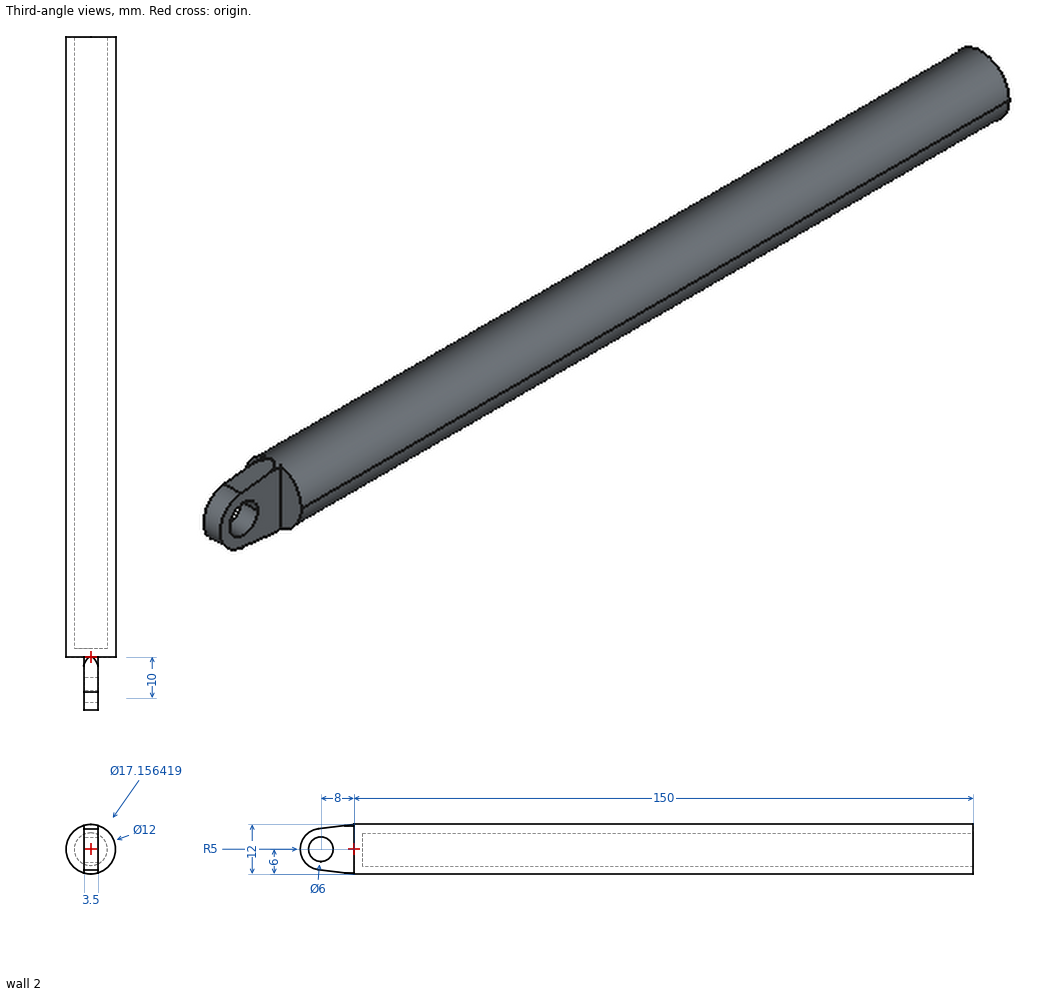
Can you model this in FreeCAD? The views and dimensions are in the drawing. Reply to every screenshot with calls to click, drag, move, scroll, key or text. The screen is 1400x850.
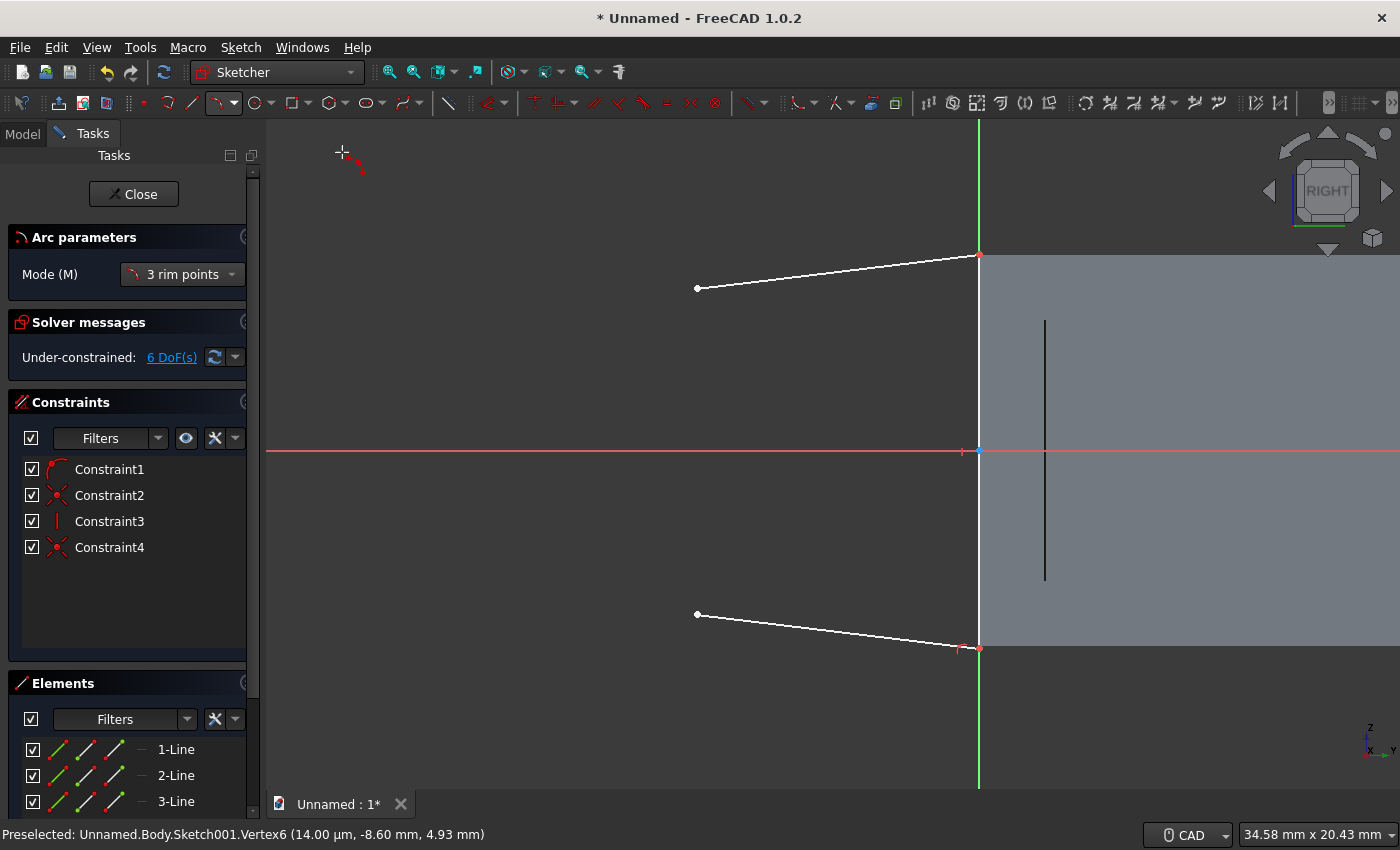
click(697, 289)
click(697, 615)
click(560, 404)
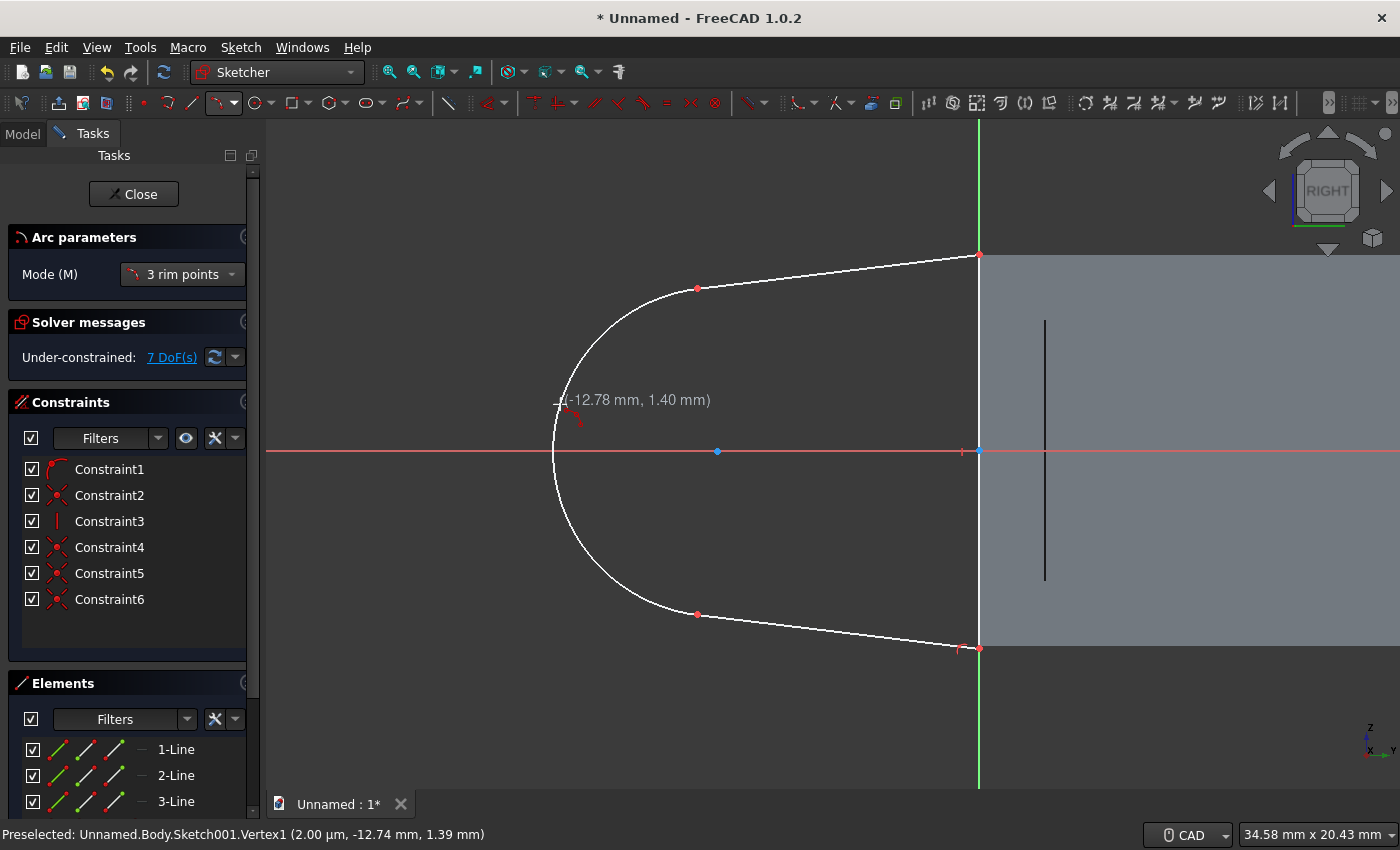
click(256, 104)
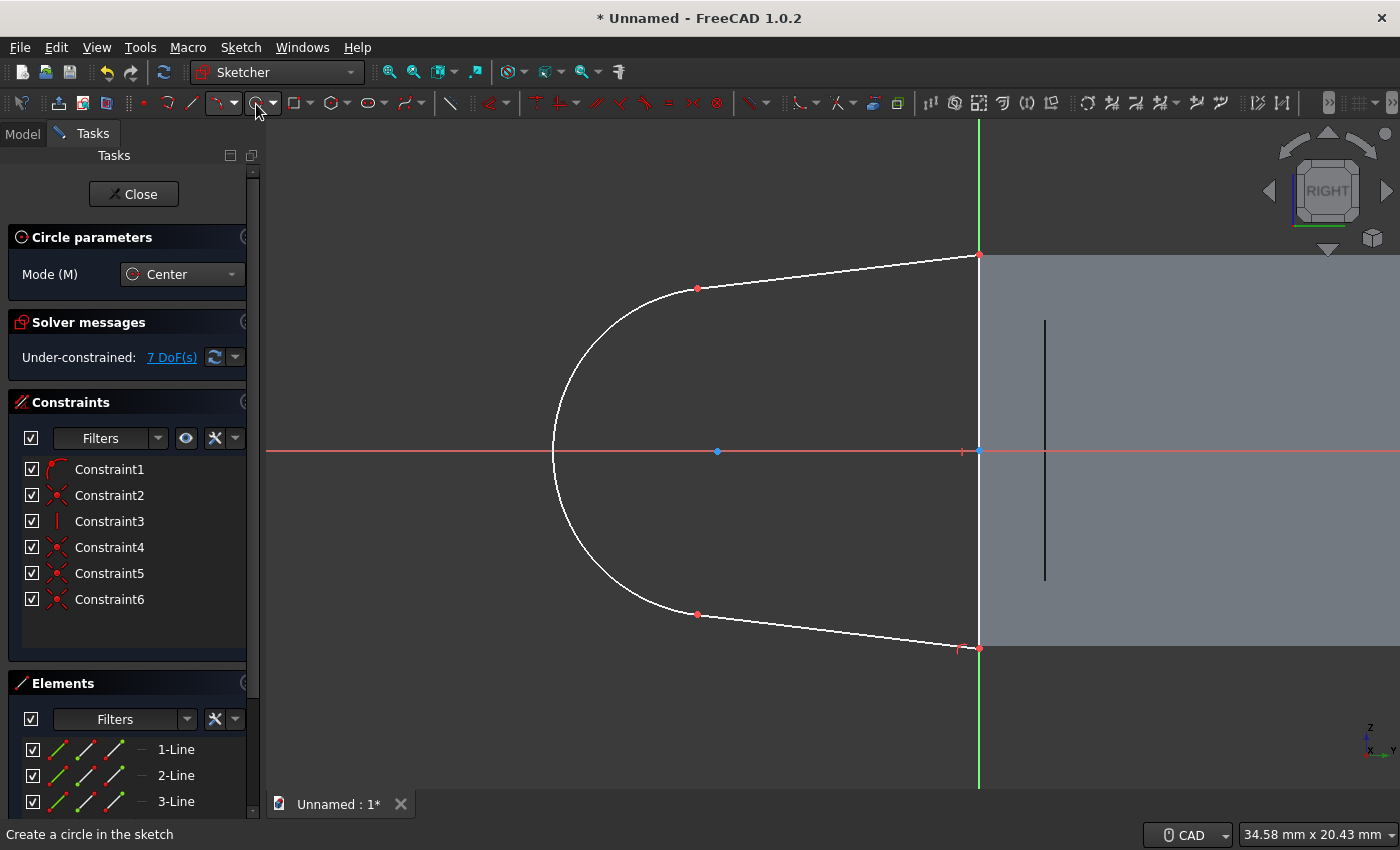
click(717, 451)
click(786, 381)
key(Escape)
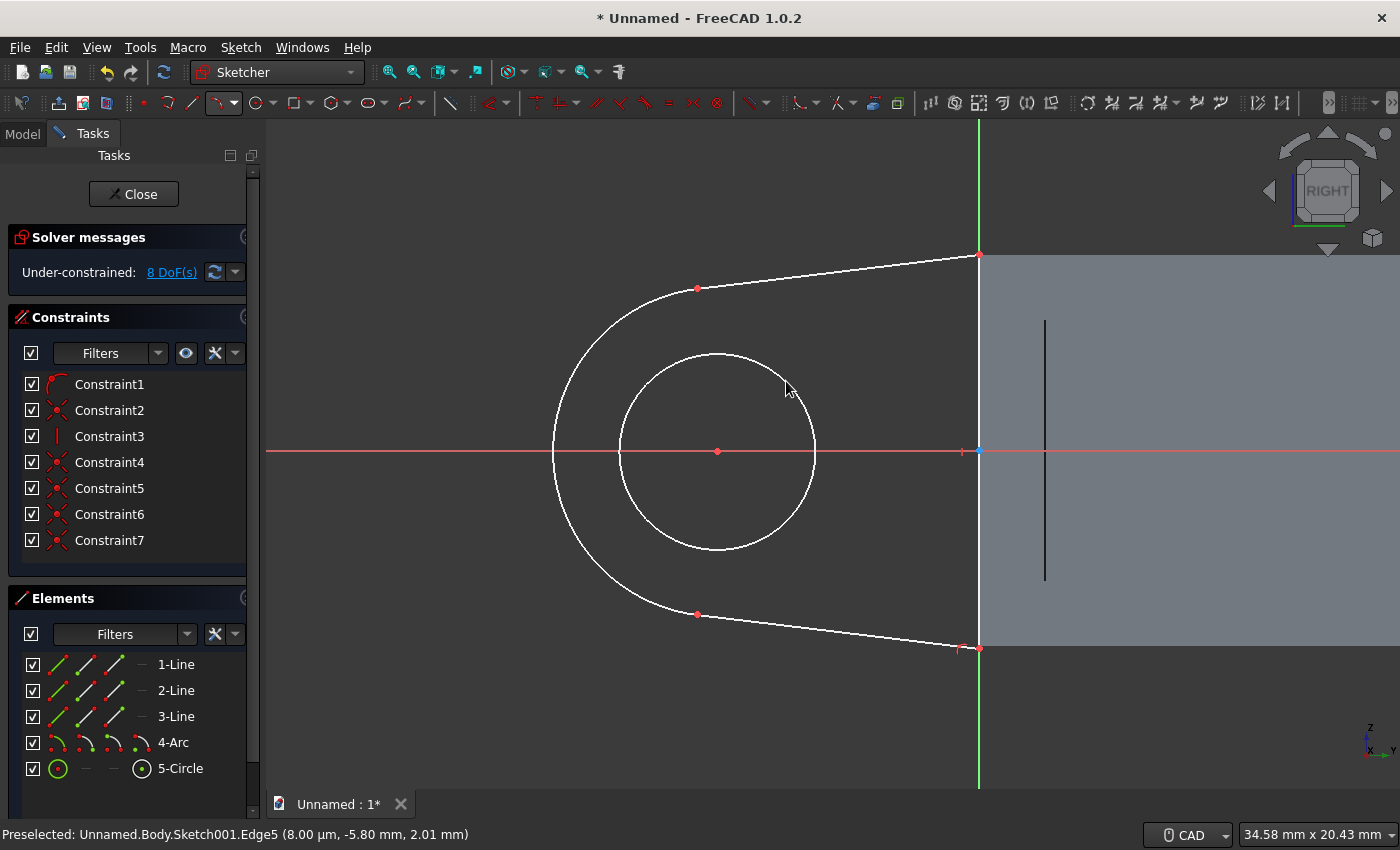
click(782, 625)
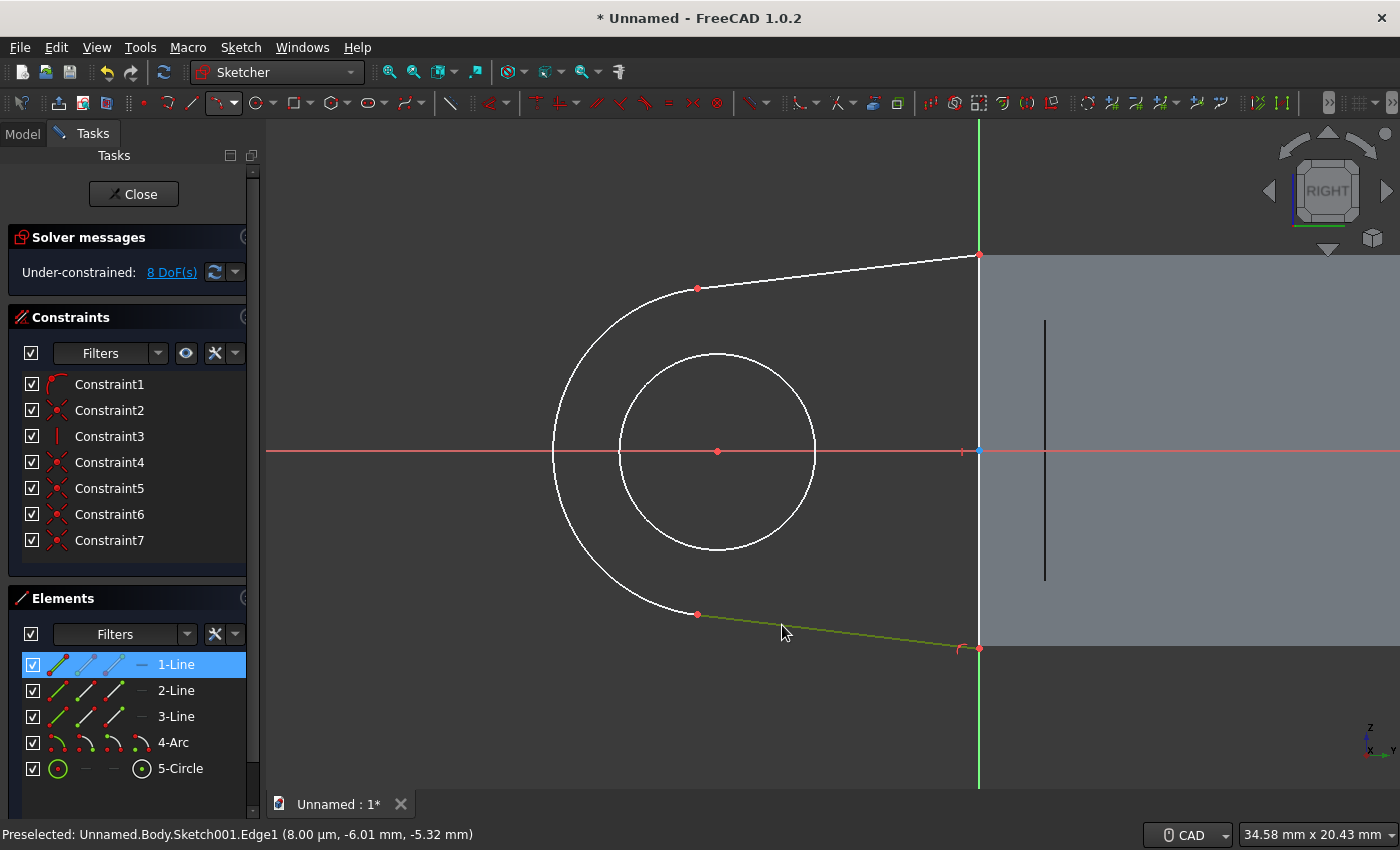
click(580, 362)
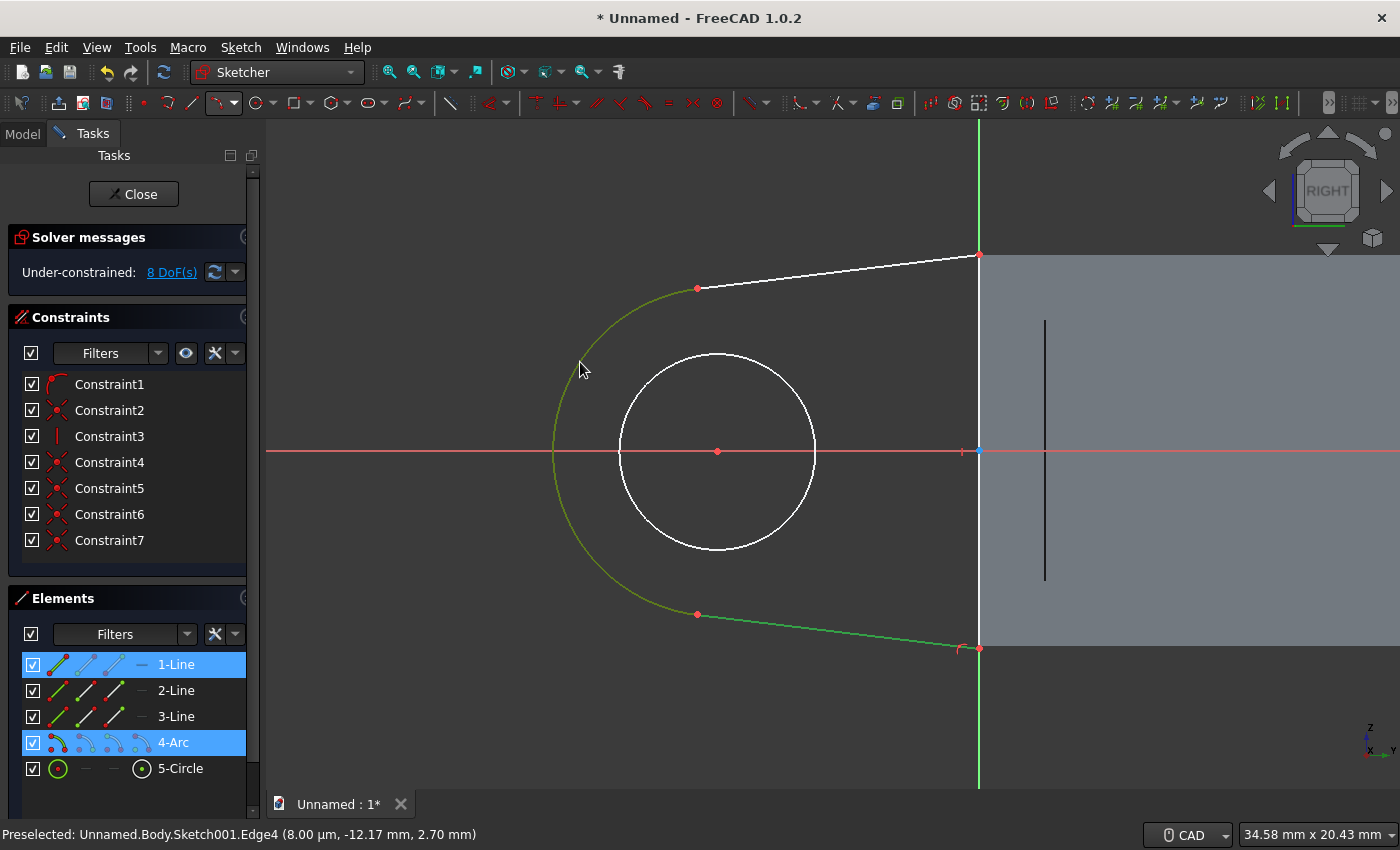
click(646, 104)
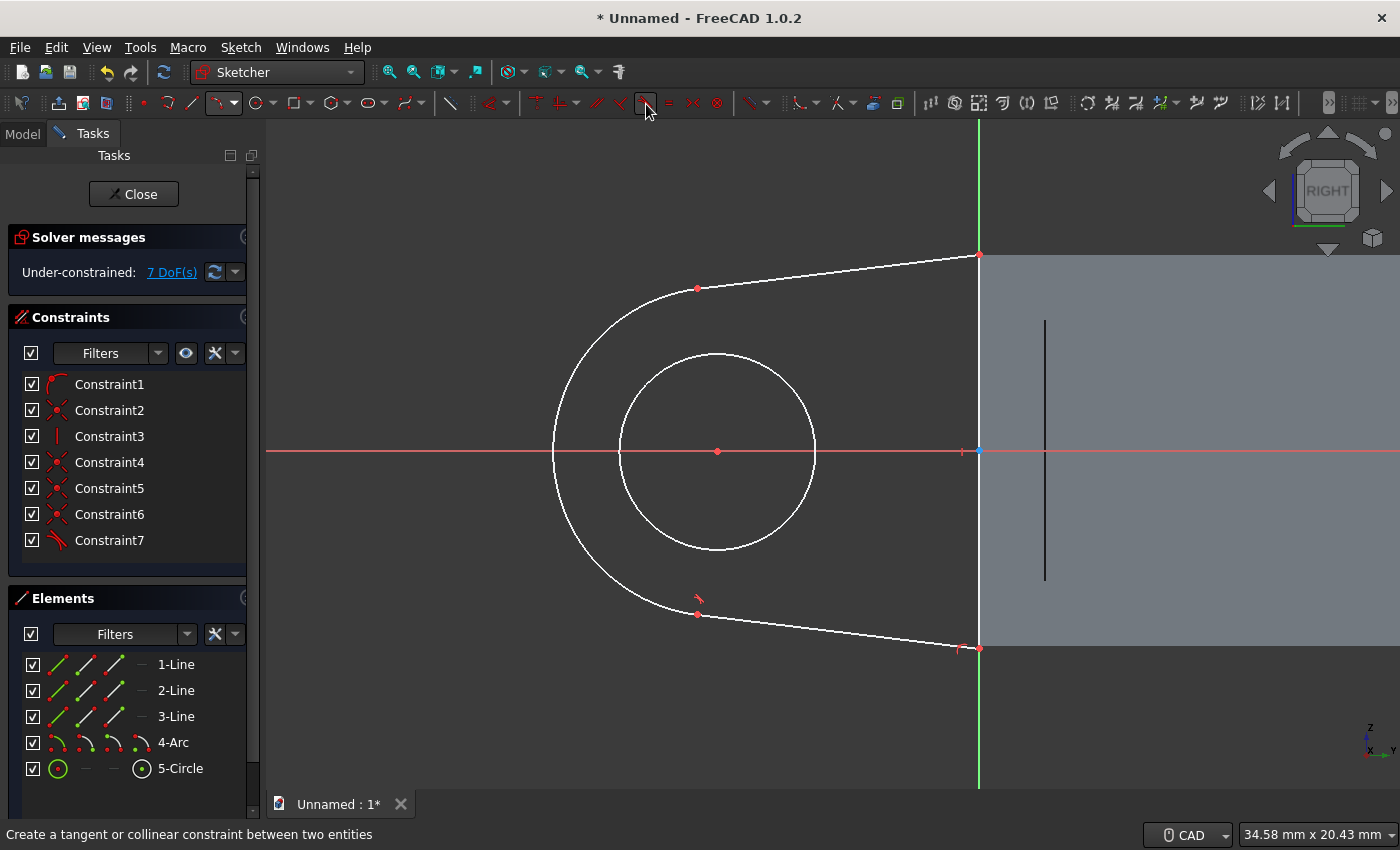
click(894, 265)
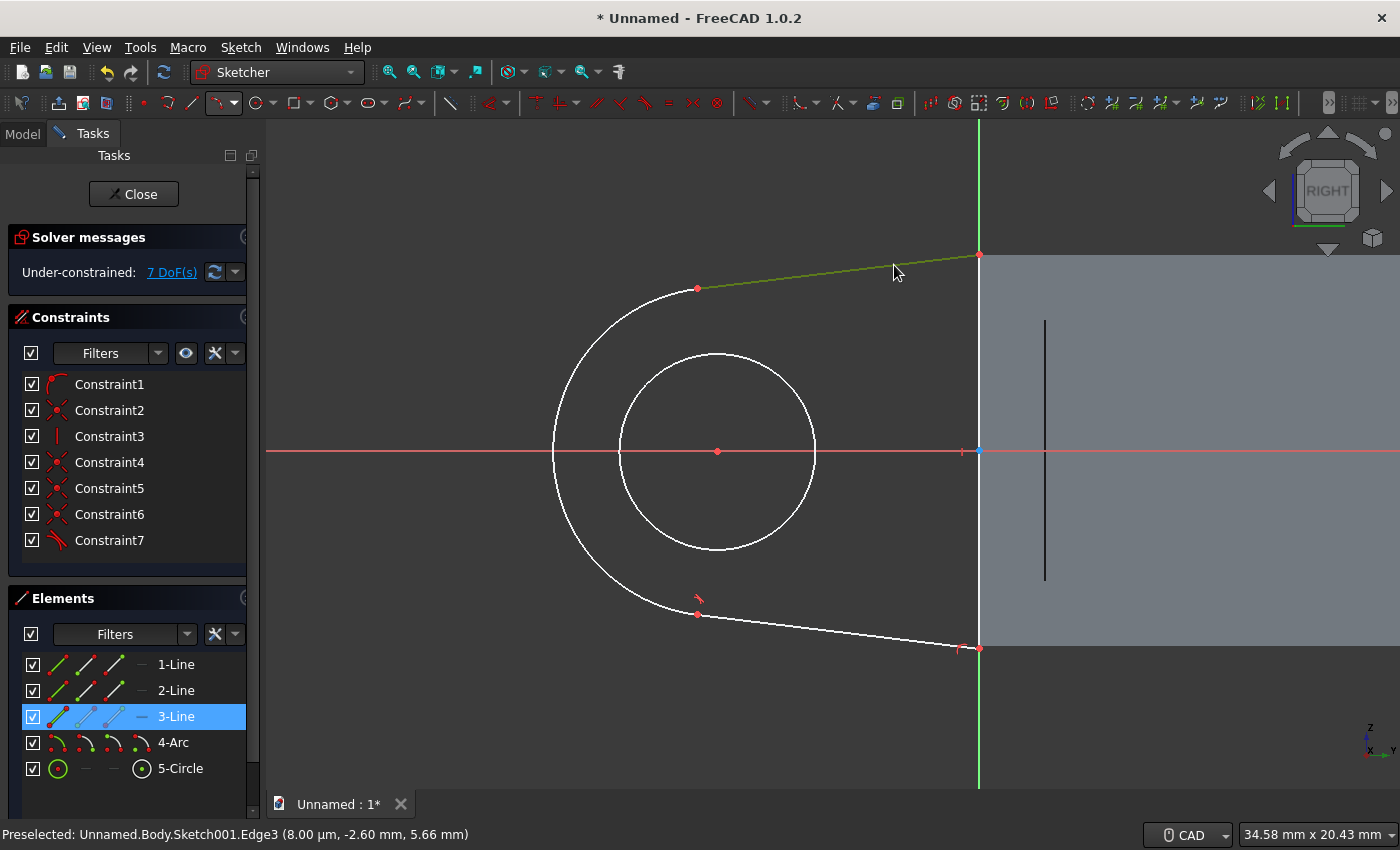
click(580, 362)